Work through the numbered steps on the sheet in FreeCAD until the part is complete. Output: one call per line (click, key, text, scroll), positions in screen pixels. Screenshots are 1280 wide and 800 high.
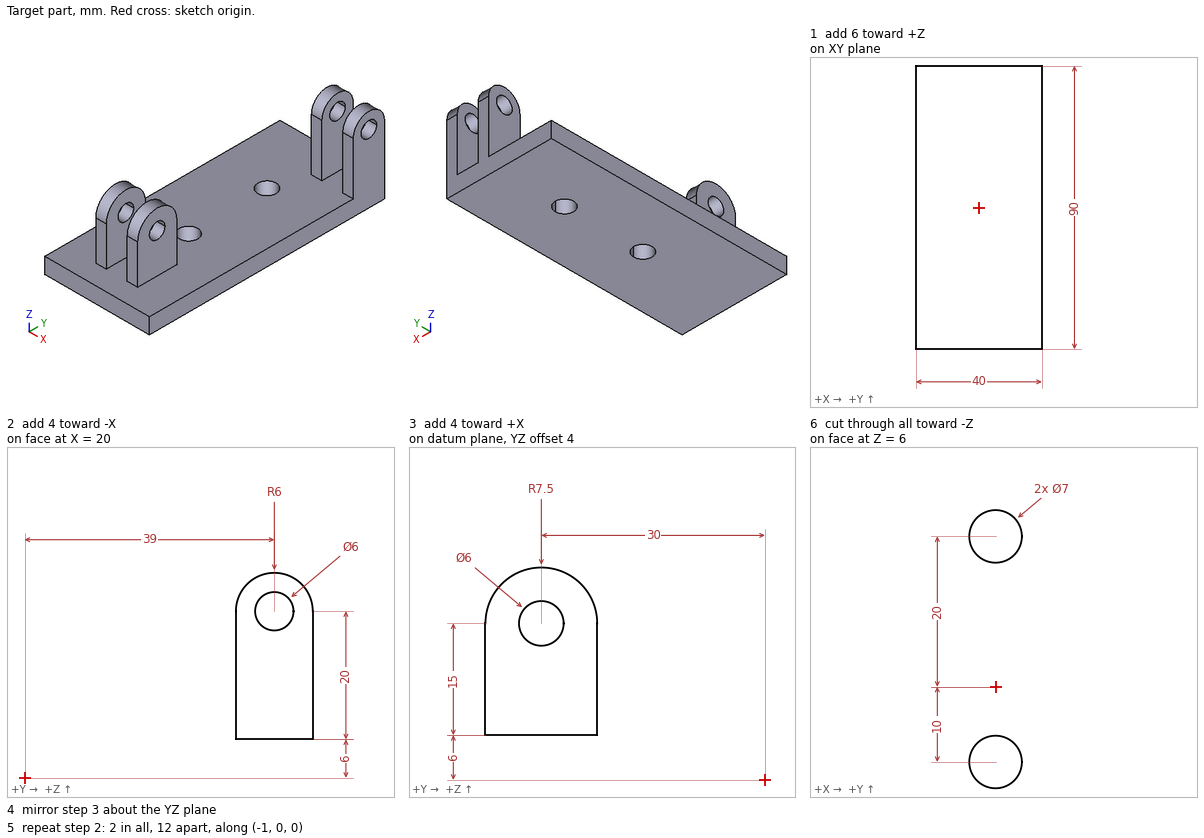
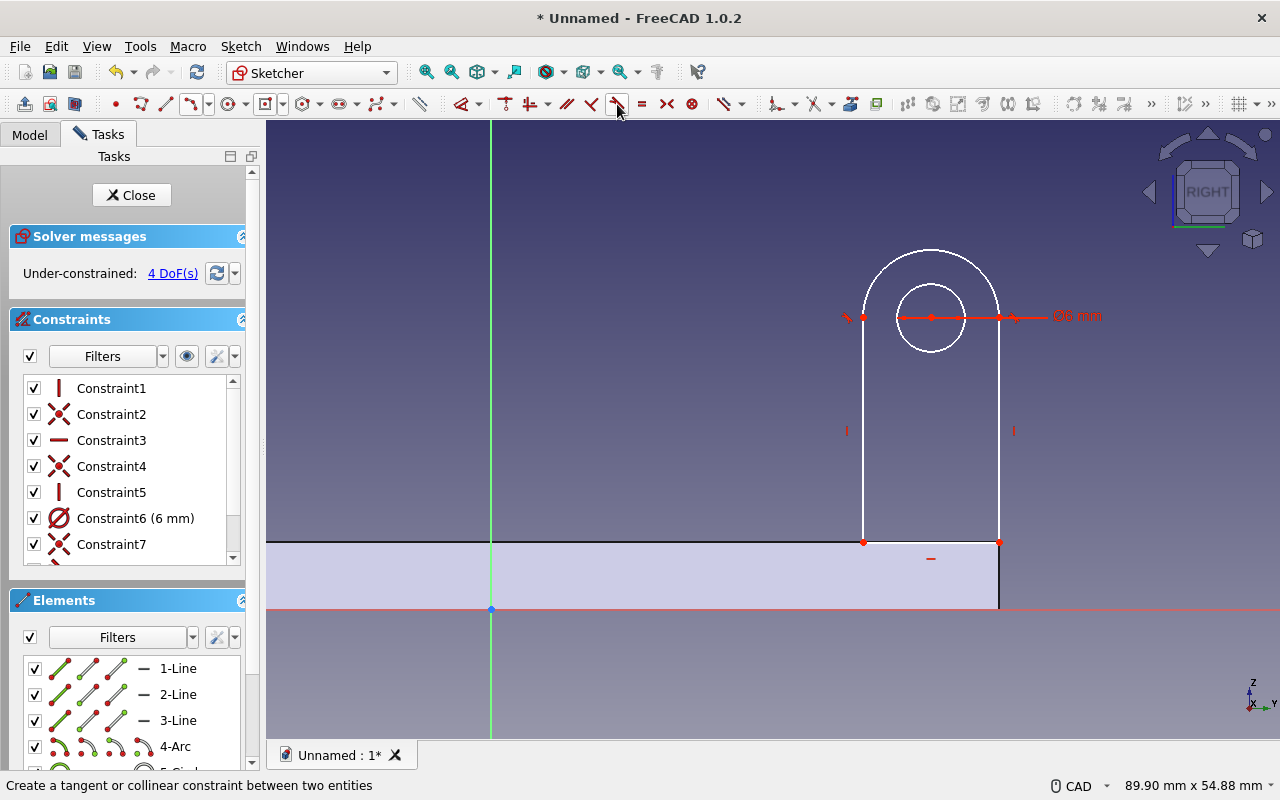
click(460, 104)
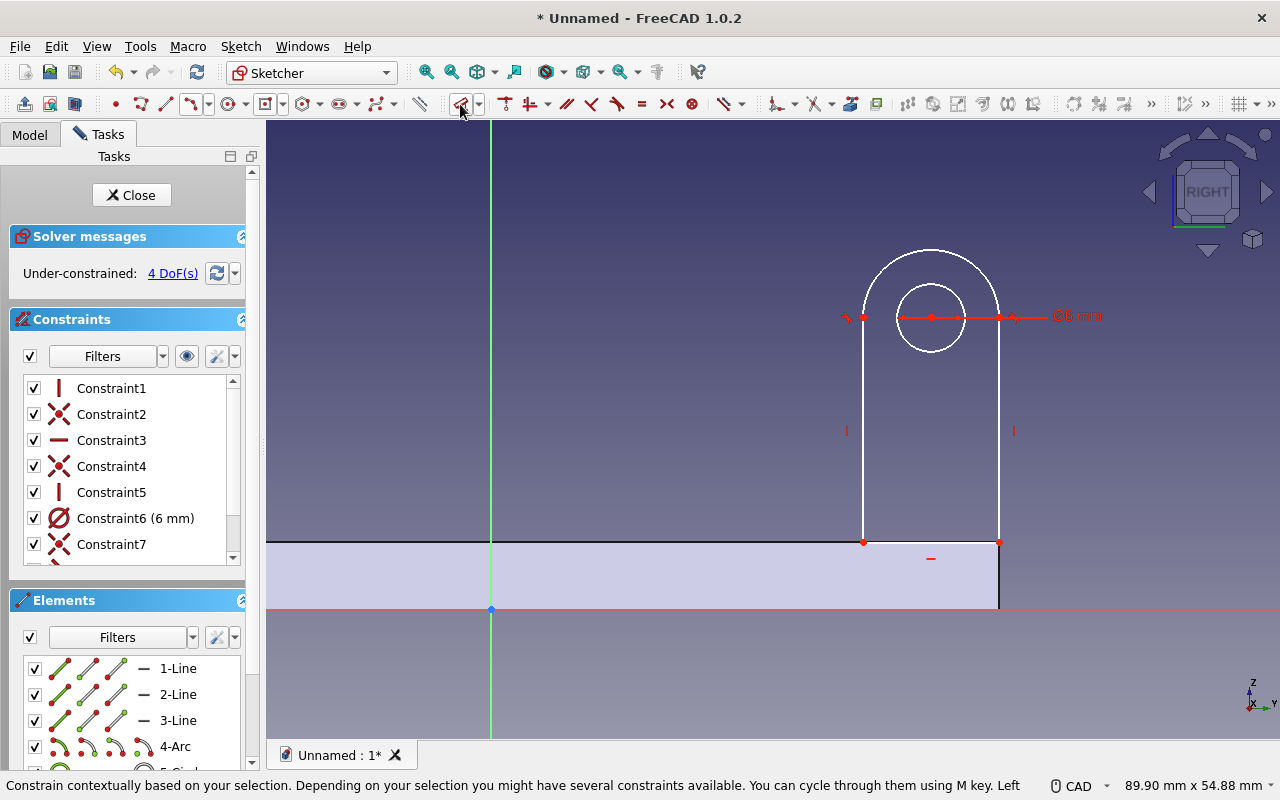
click(971, 263)
click(990, 237)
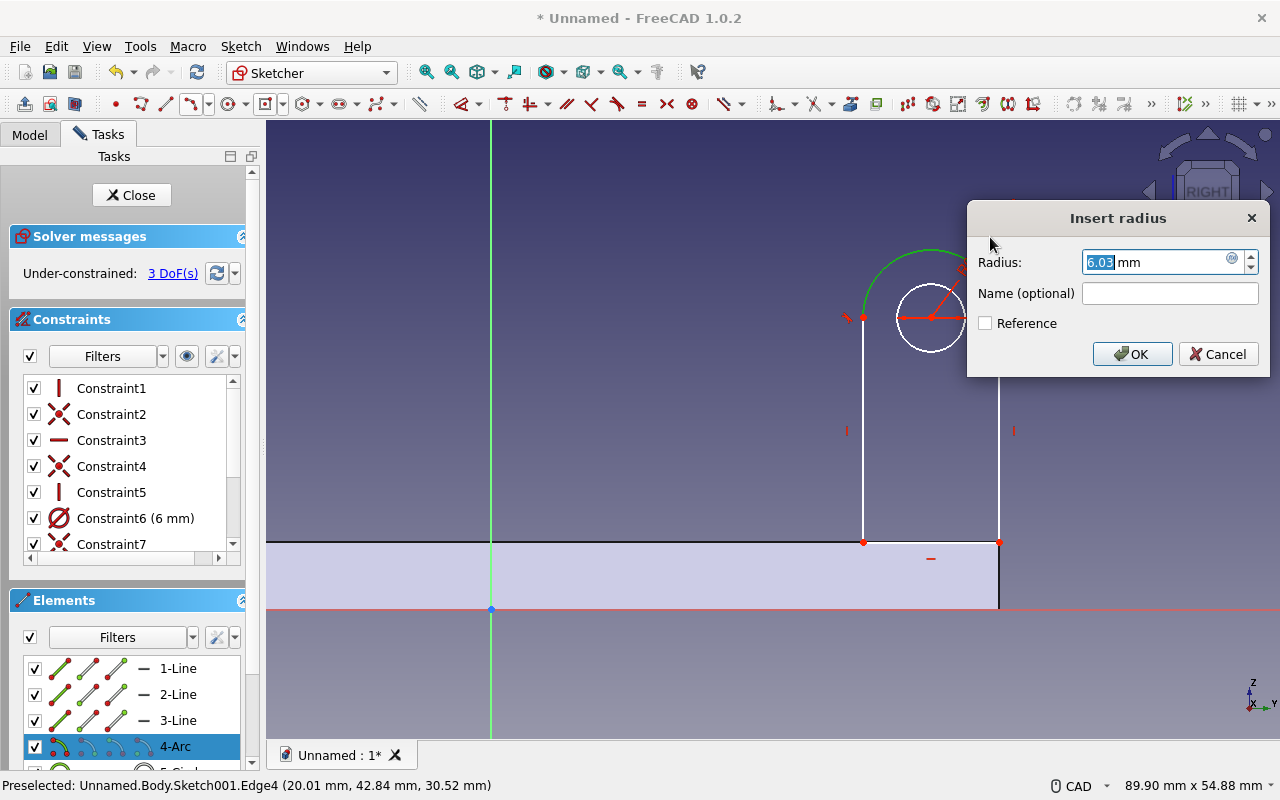
text(6)
key(Return)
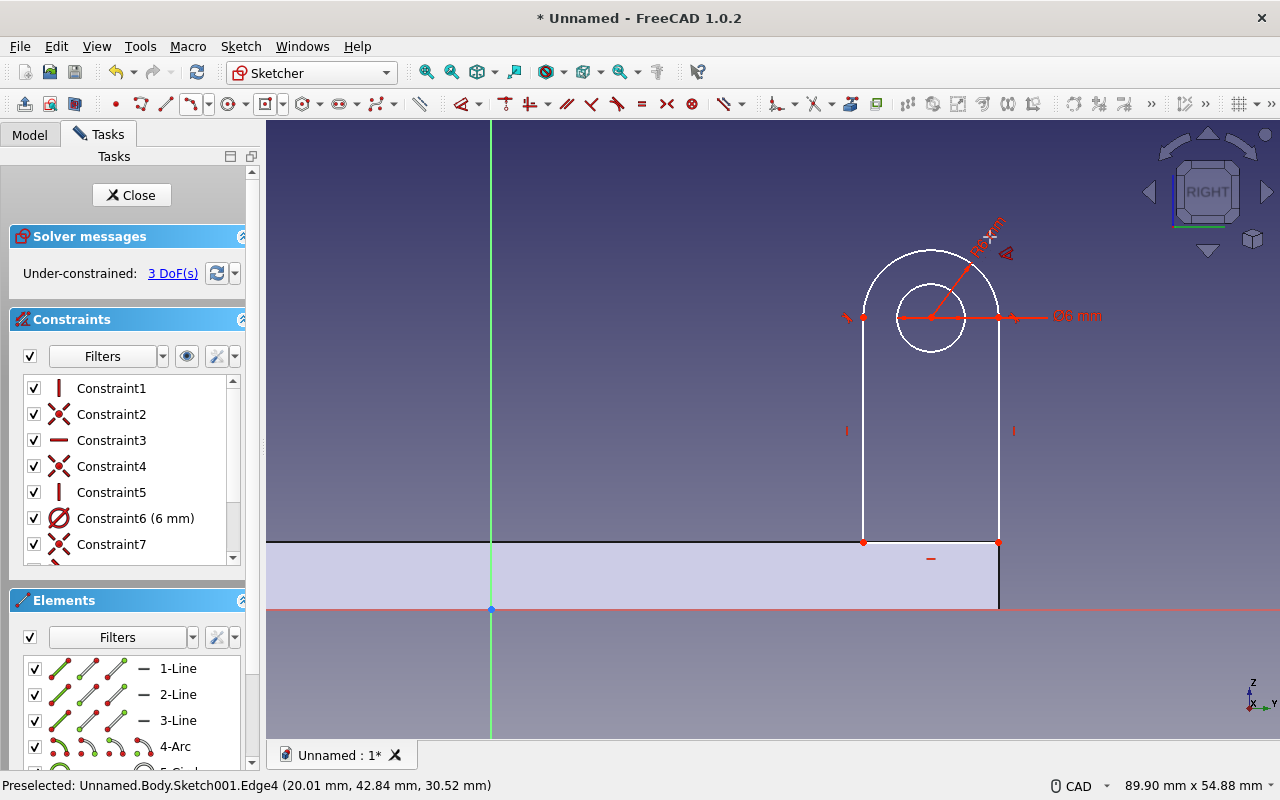
click(999, 385)
click(1033, 430)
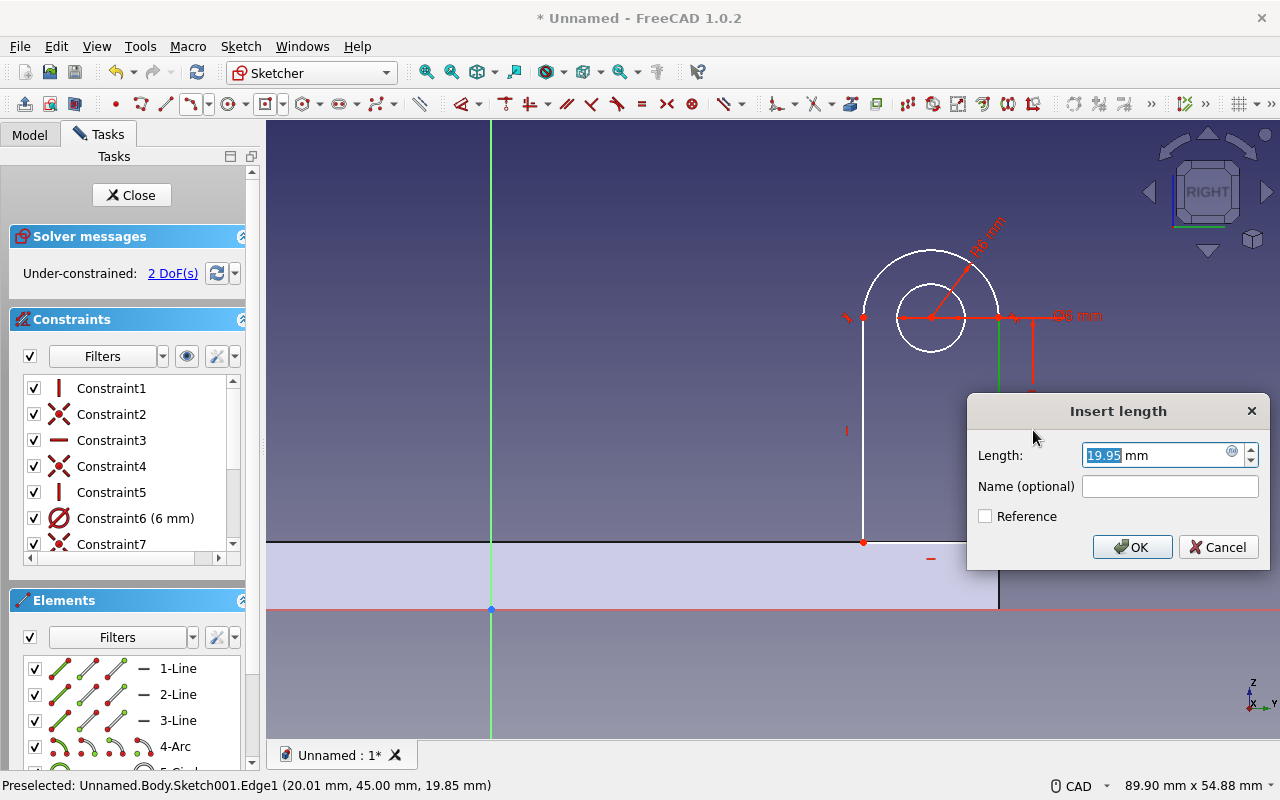
text(20)
key(Return)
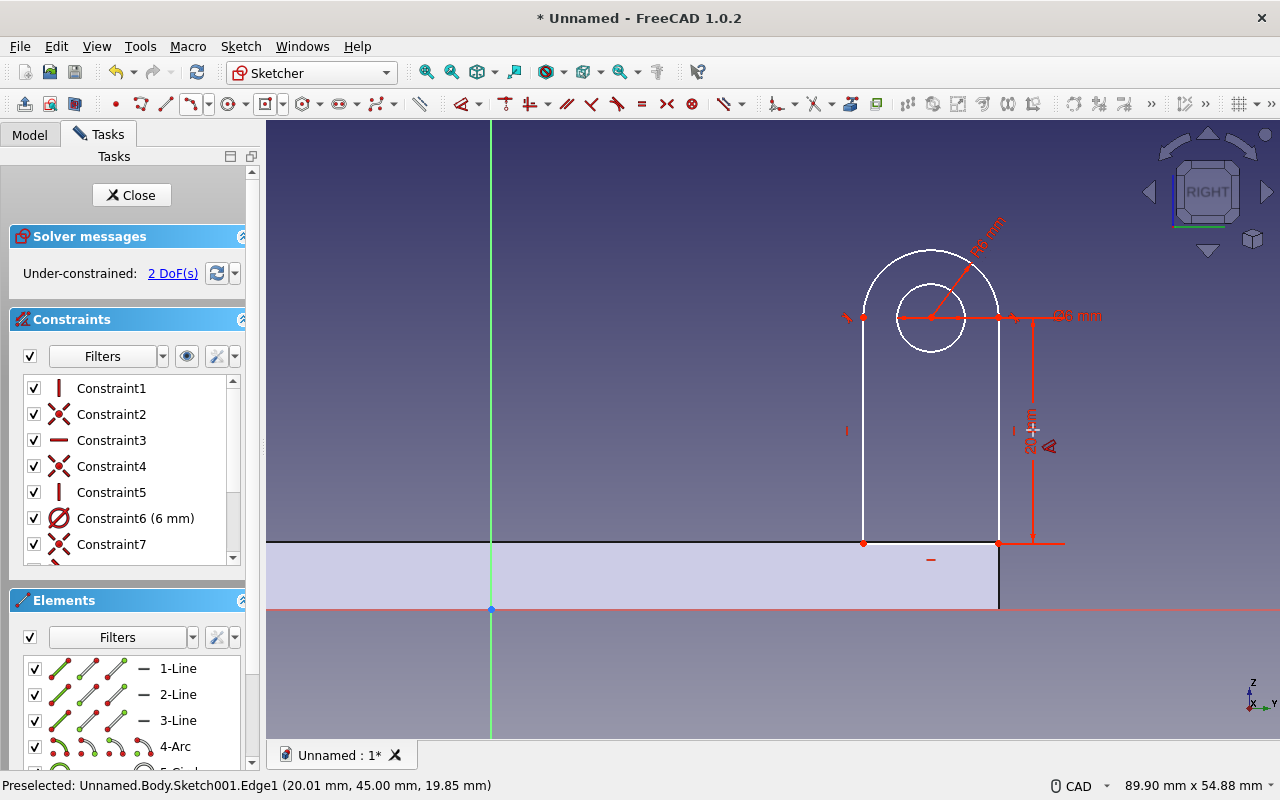
click(999, 544)
click(457, 577)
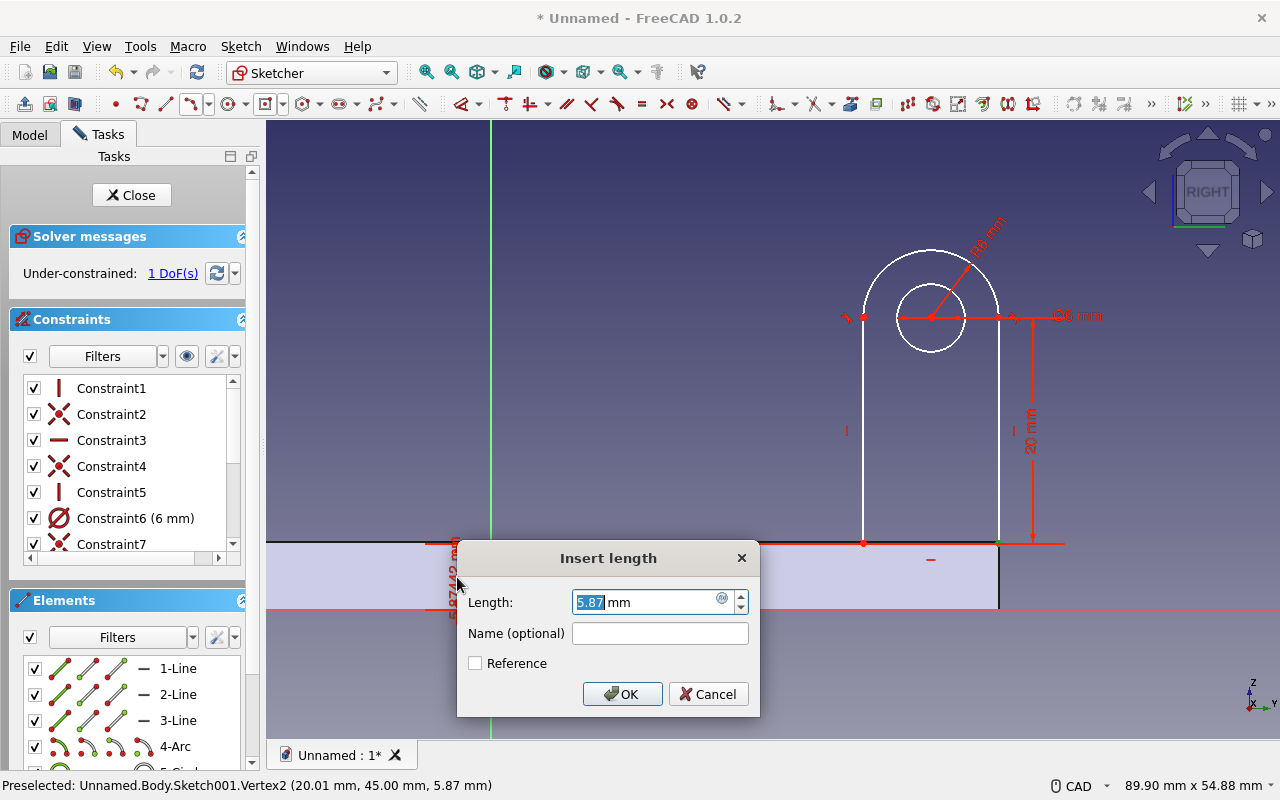
text(6)
key(Return)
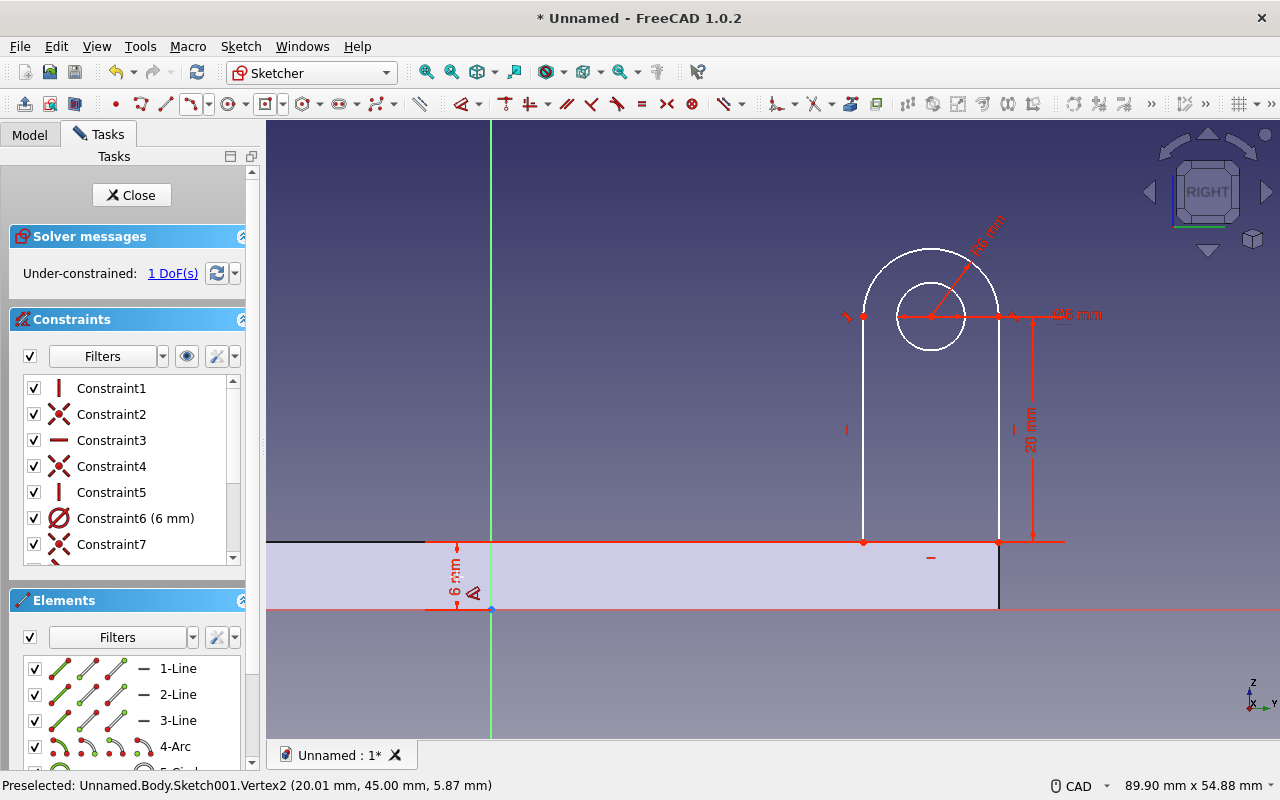
click(931, 317)
click(711, 644)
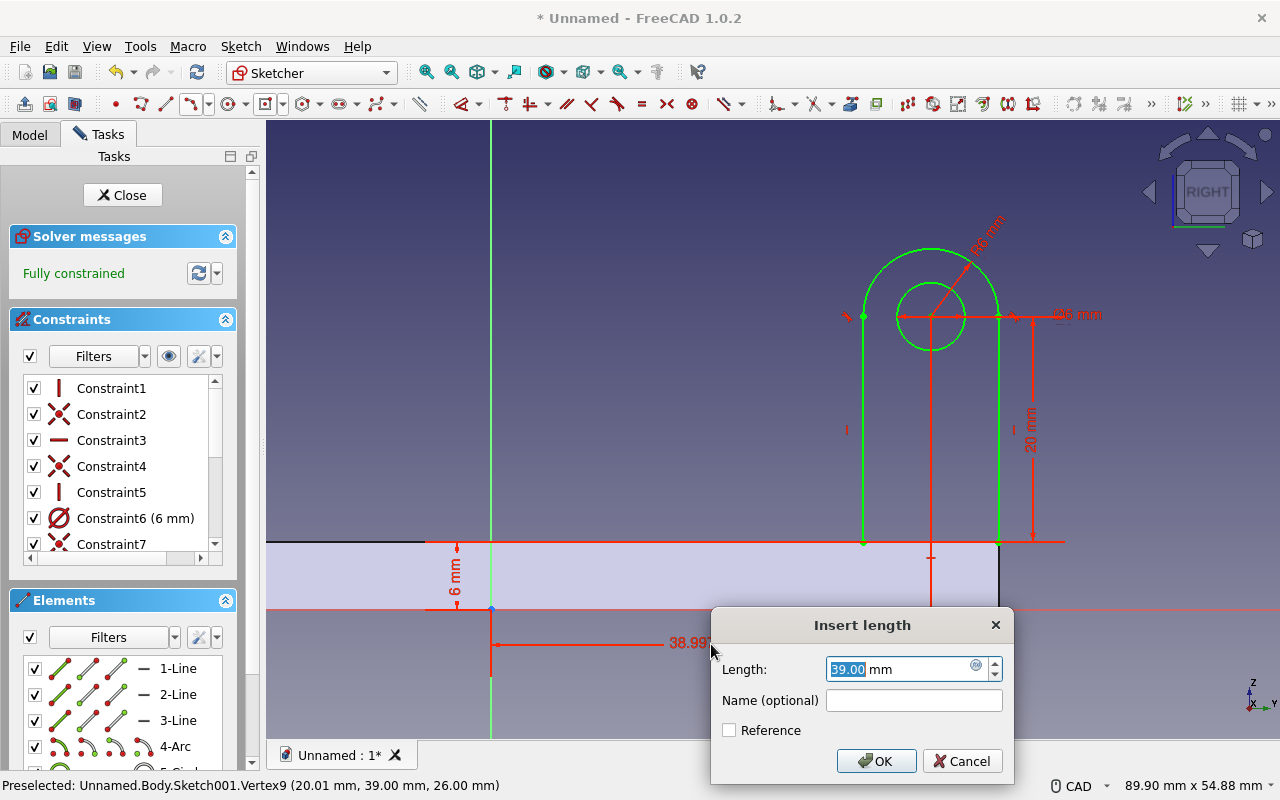
text(39)
key(Return)
key(Escape)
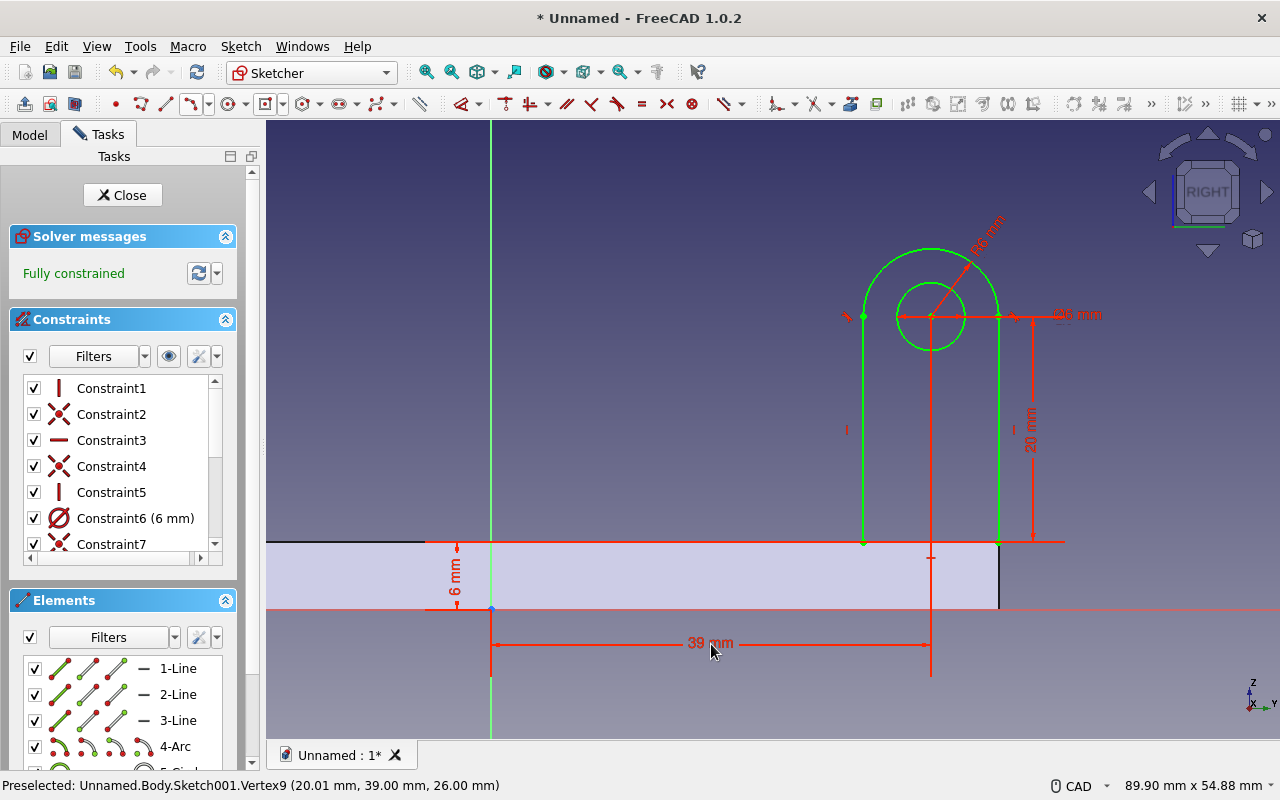
click(123, 195)